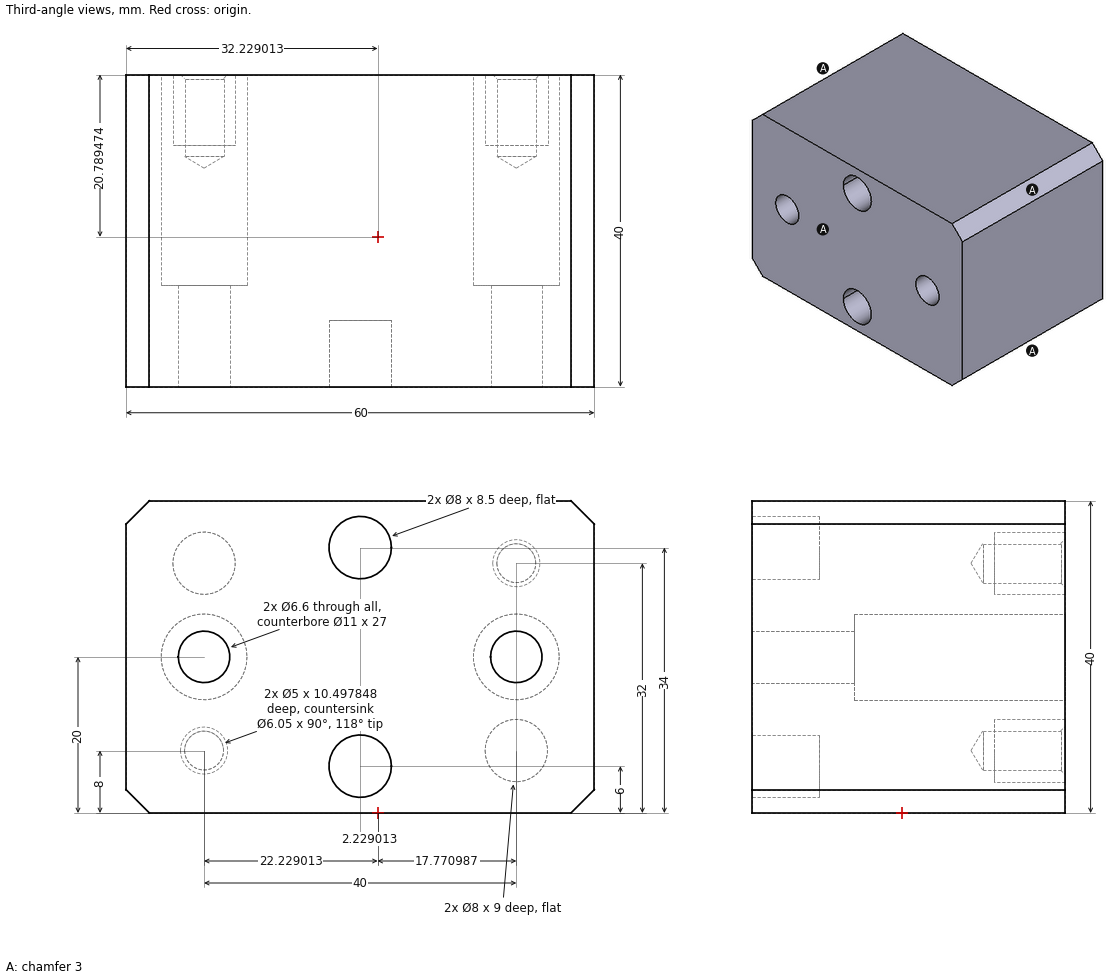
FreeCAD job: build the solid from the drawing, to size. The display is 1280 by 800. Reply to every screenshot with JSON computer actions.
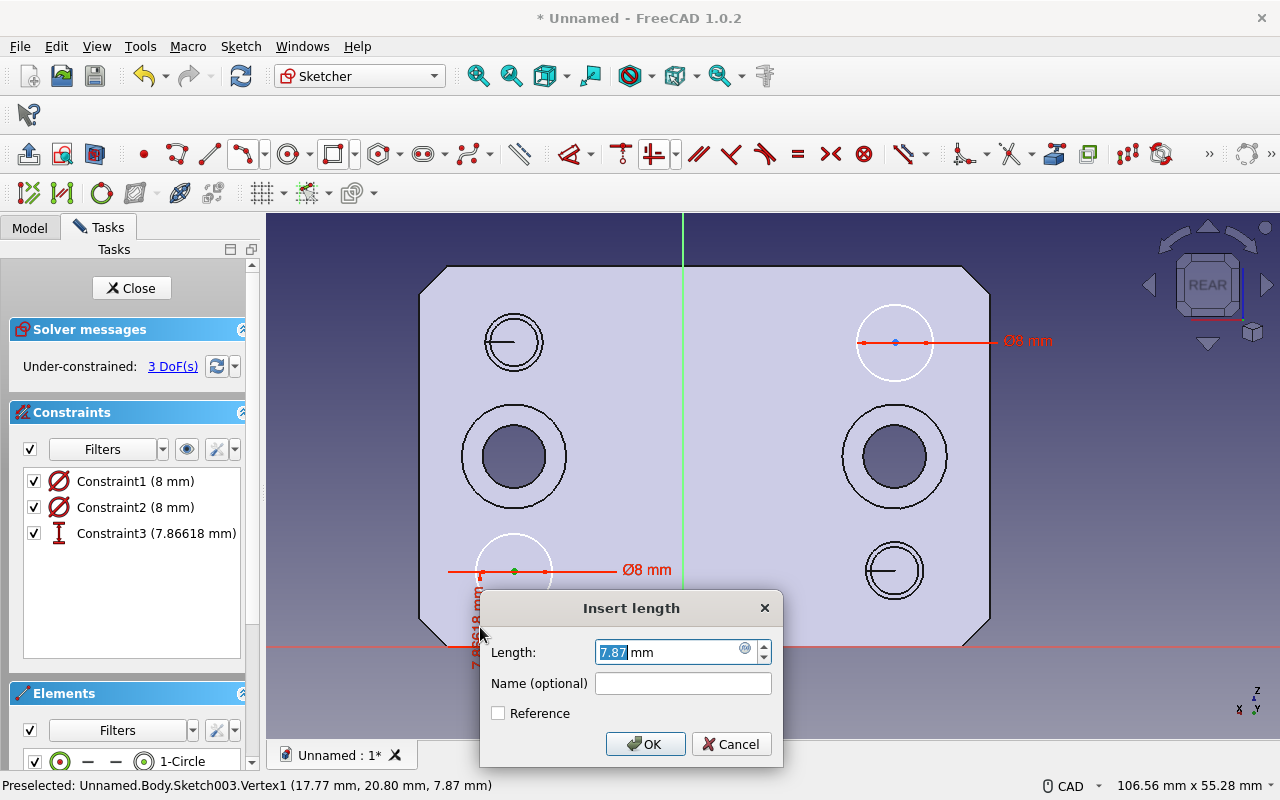
{"action": "type", "text": "8"}
{"action": "key", "text": "Return"}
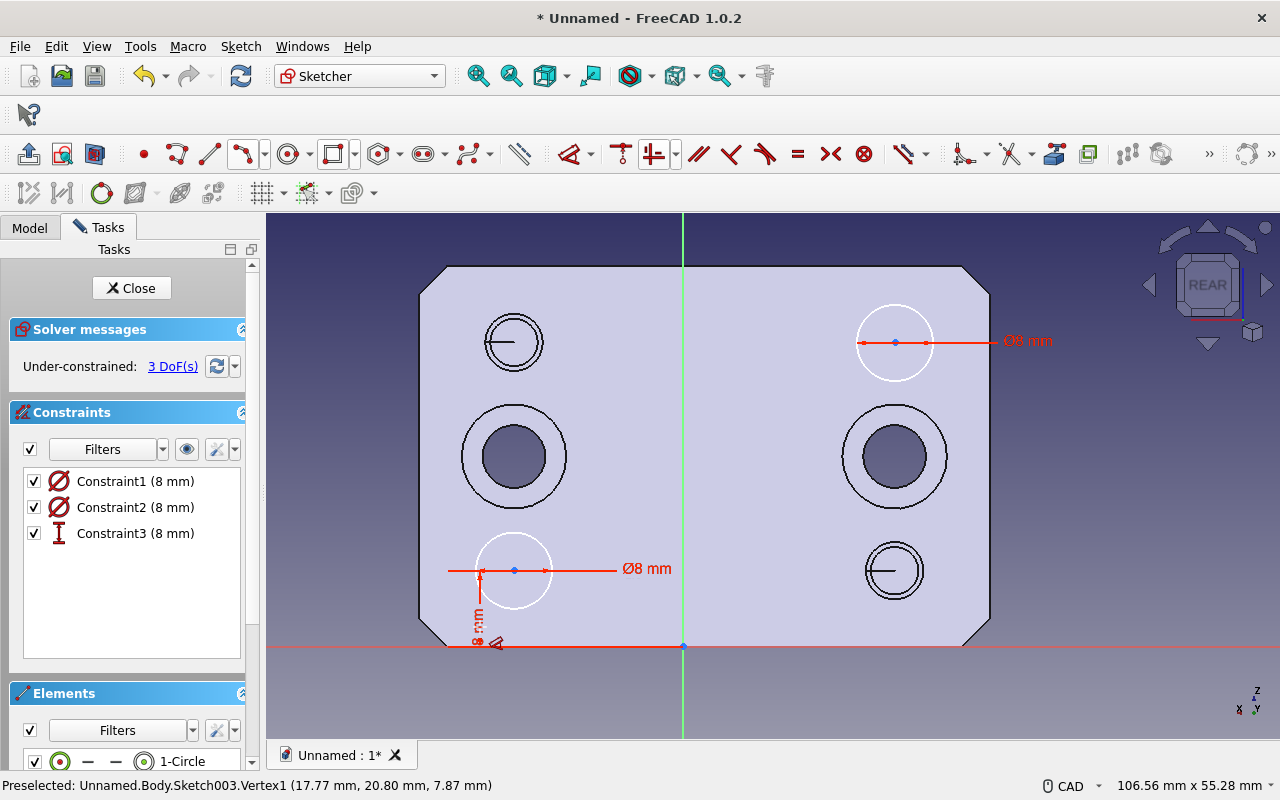
{"action": "left_click", "coordinate": [895, 343]}
{"action": "left_click", "coordinate": [929, 495]}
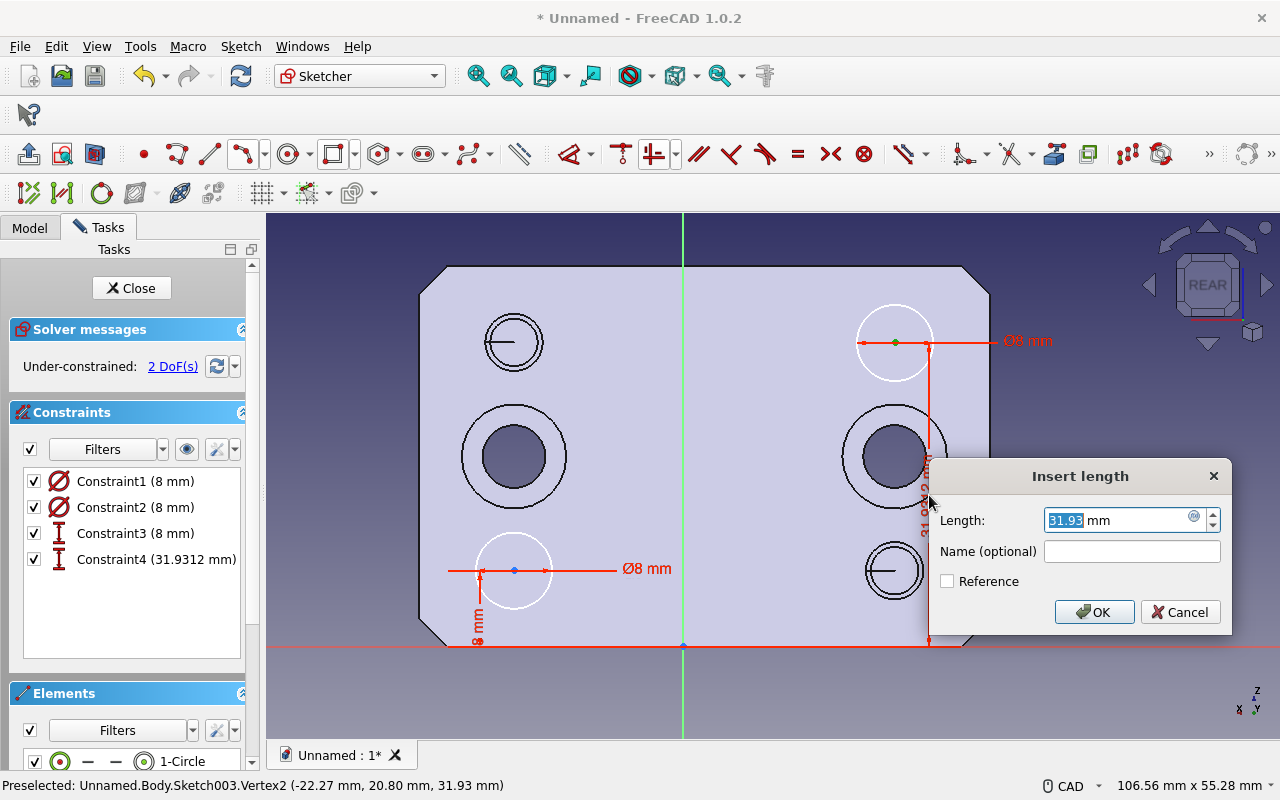
{"action": "type", "text": "32"}
{"action": "key", "text": "Return"}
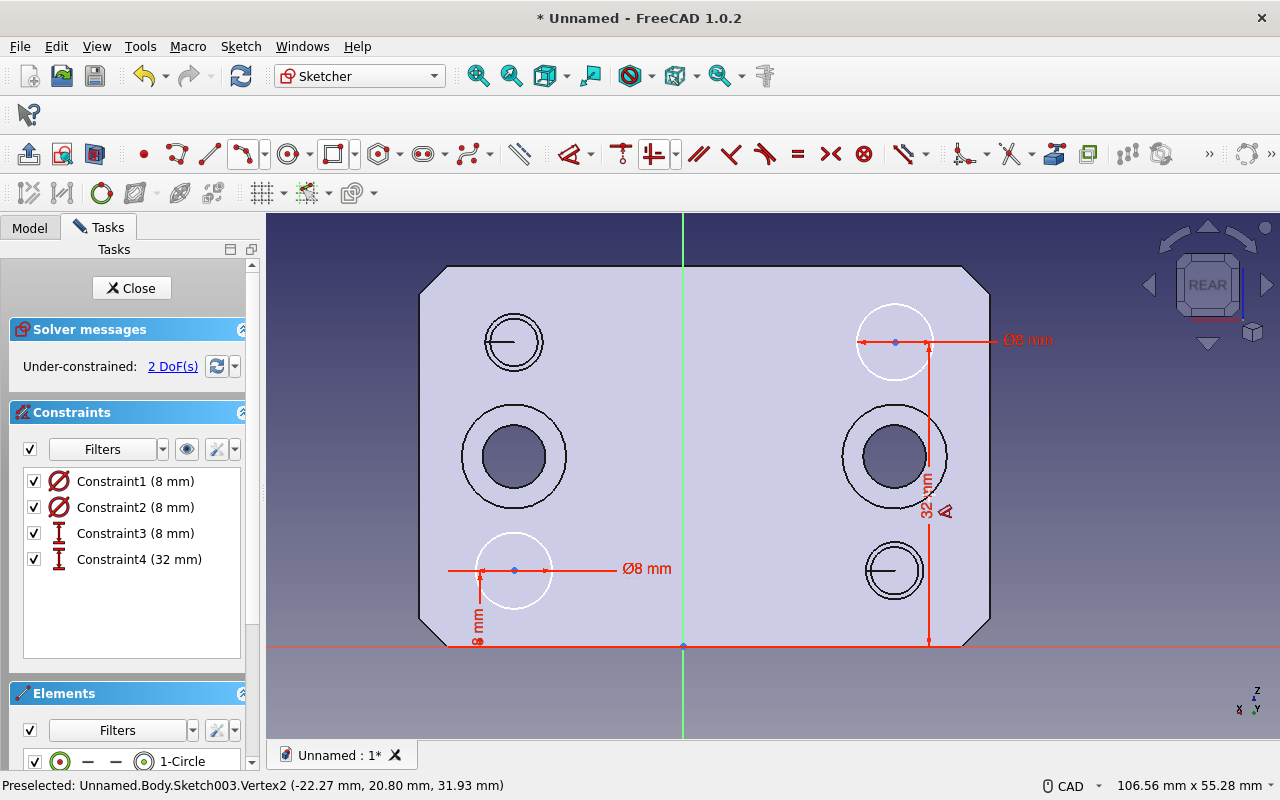
{"action": "left_click", "coordinate": [514, 571]}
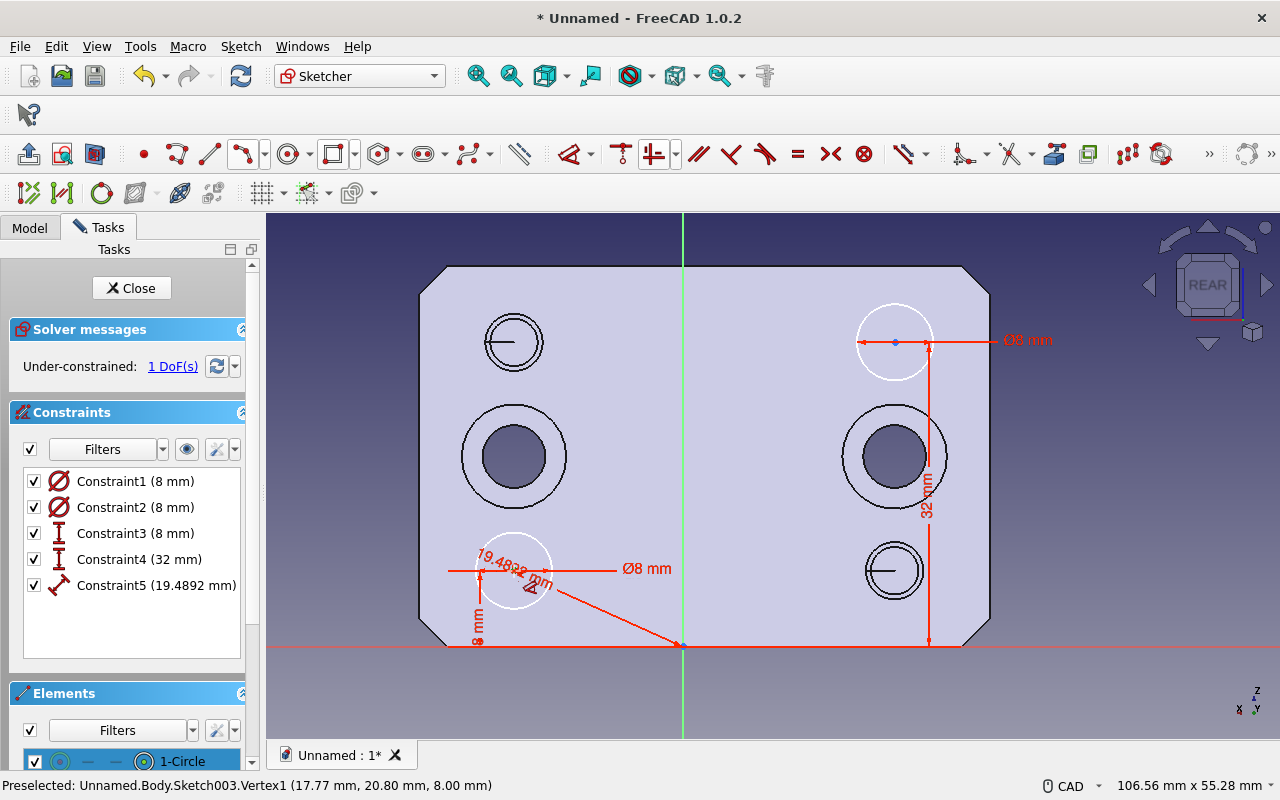
{"action": "left_click", "coordinate": [895, 342]}
{"action": "left_click", "coordinate": [704, 308]}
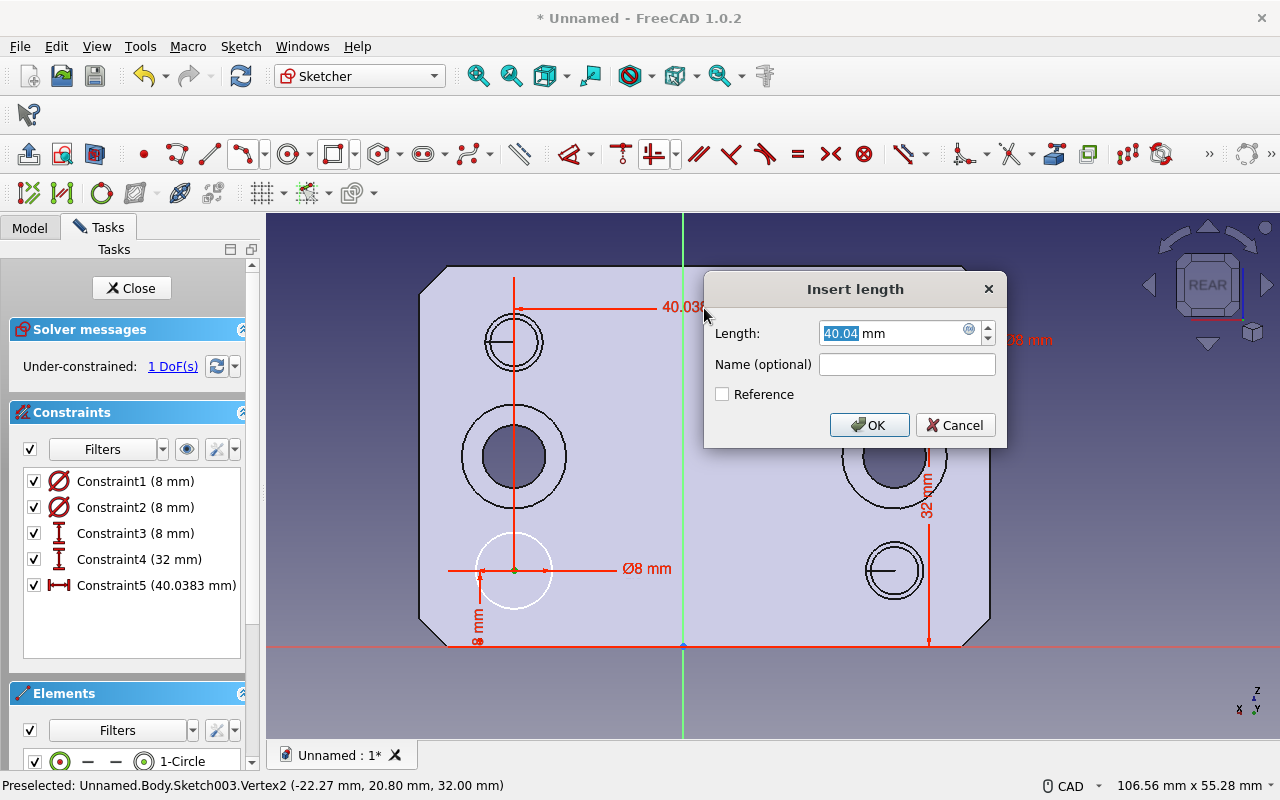
{"action": "type", "text": "40"}
{"action": "key", "text": "Return"}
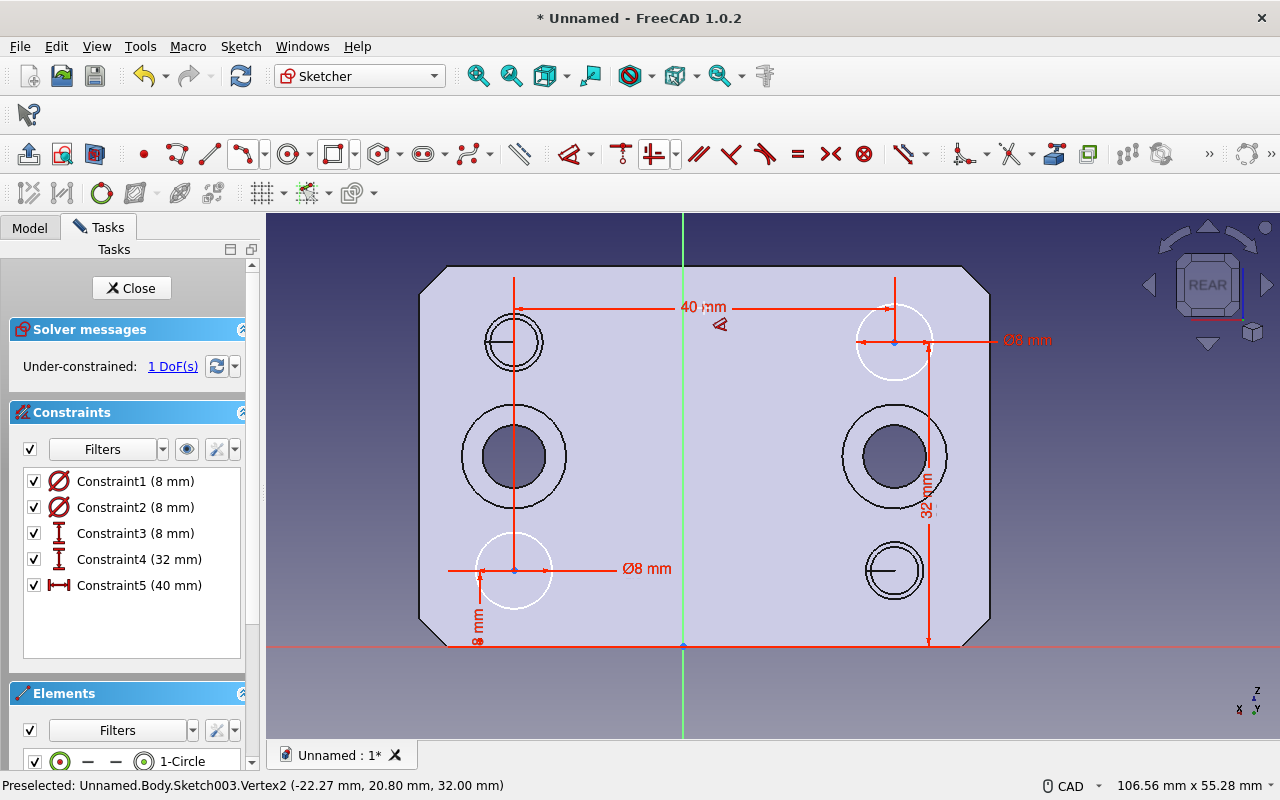
{"action": "left_click", "coordinate": [514, 571]}
{"action": "left_click", "coordinate": [599, 681]}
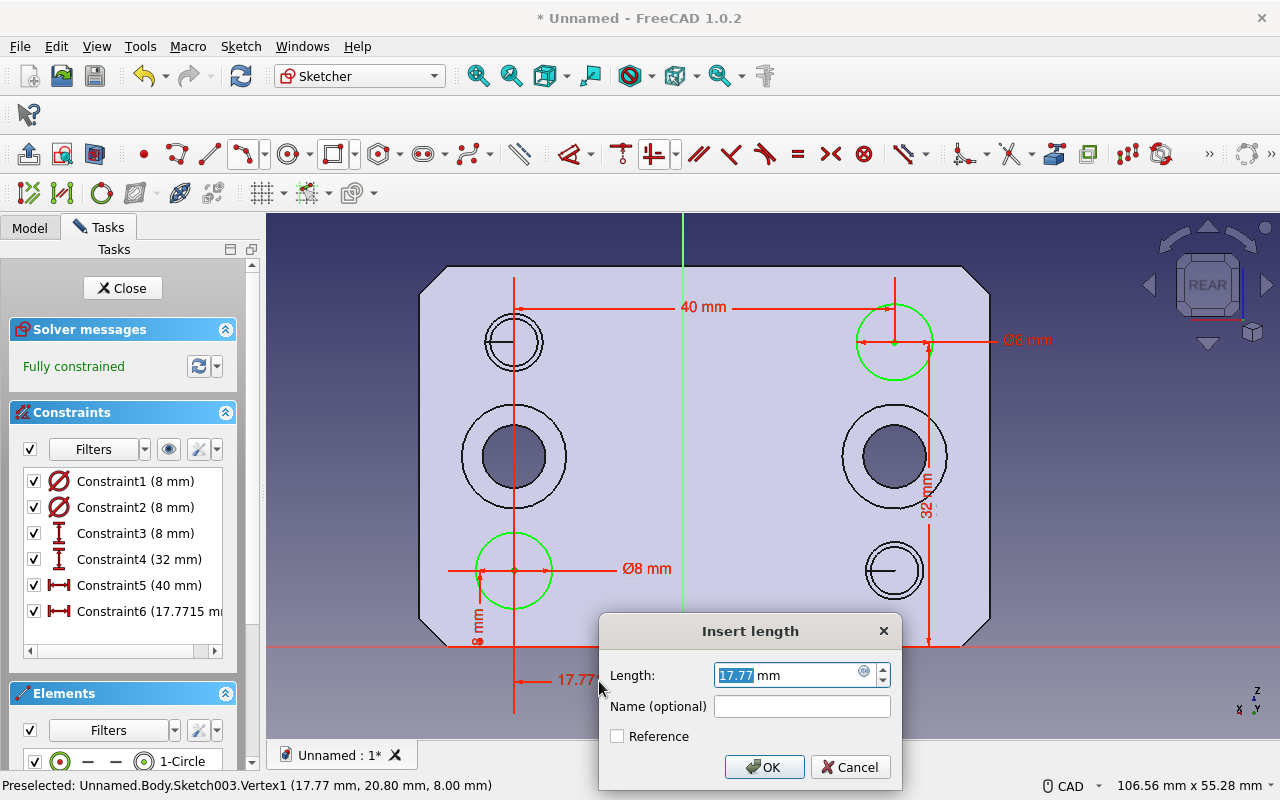
{"action": "type", "text": "17.770987"}
{"action": "key", "text": "Return"}
{"action": "key", "text": "Escape"}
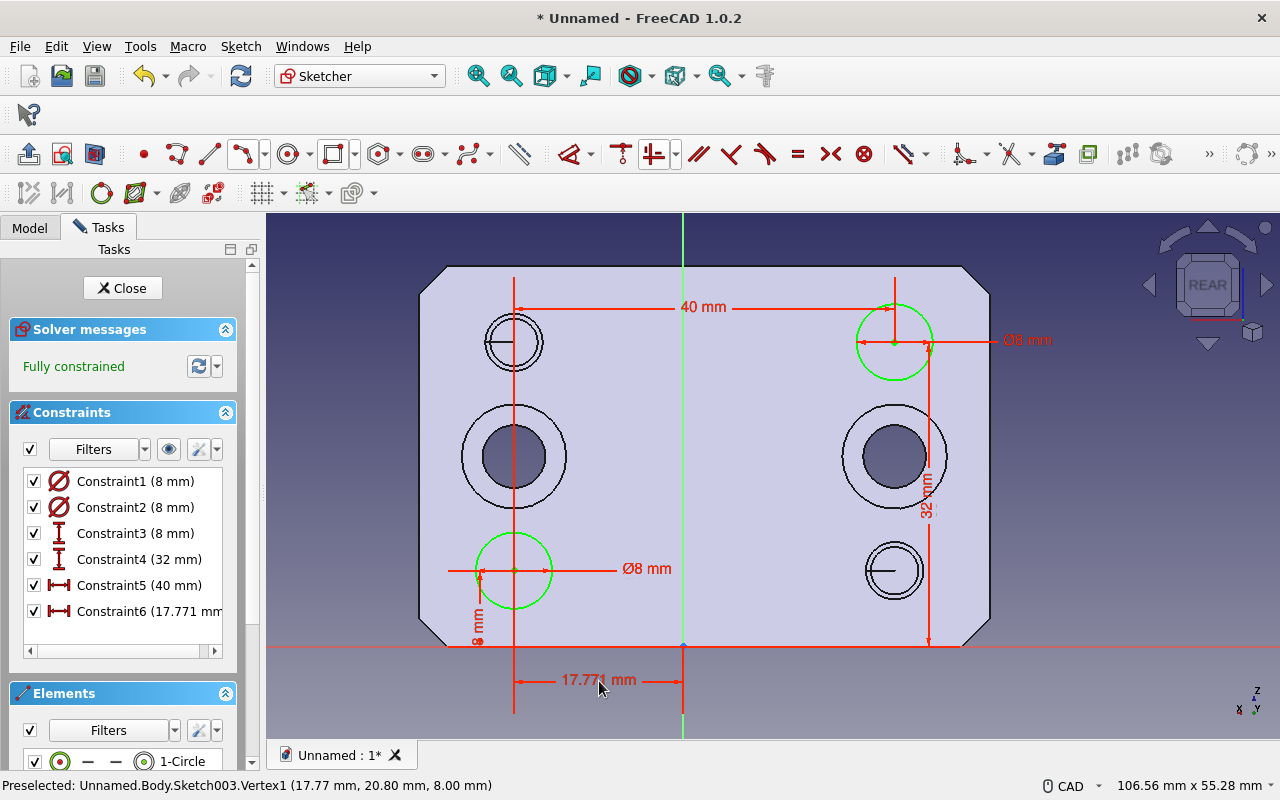
{"action": "left_click", "coordinate": [123, 288]}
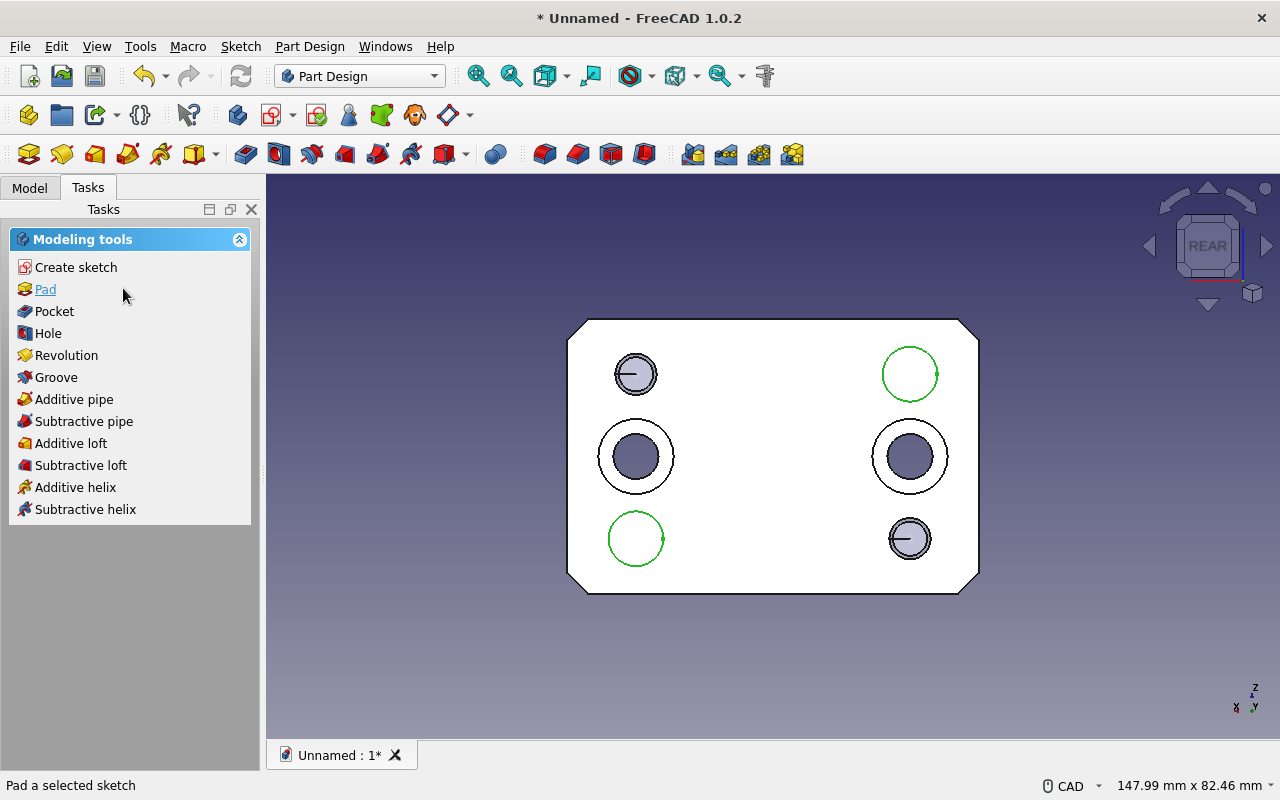
{"action": "left_click", "coordinate": [279, 154]}